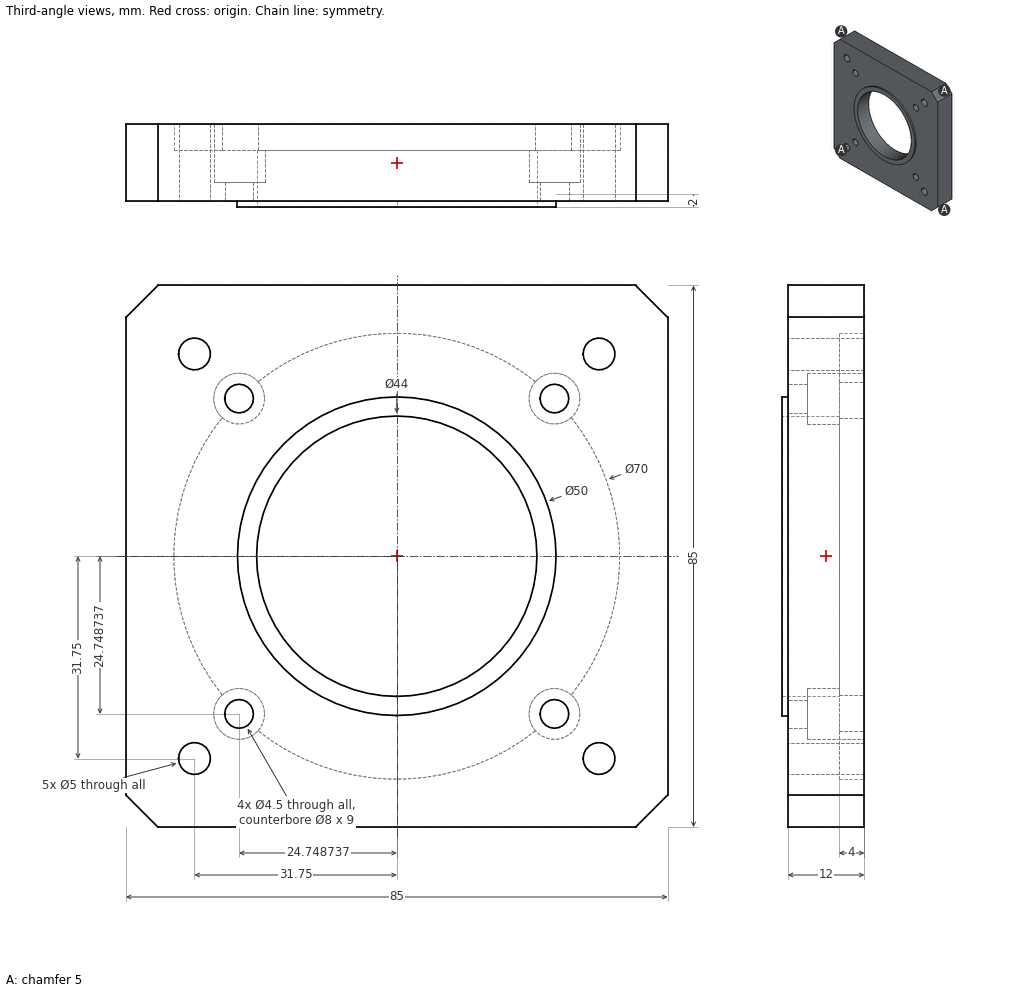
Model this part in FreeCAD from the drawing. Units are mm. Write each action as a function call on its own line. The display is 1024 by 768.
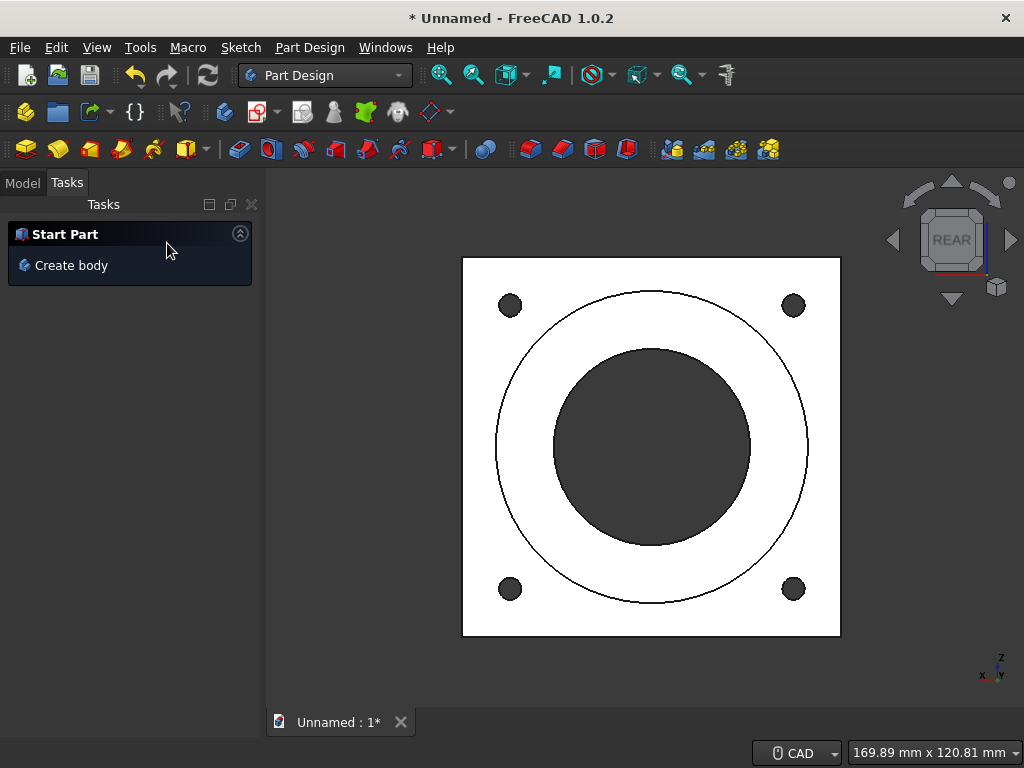
key(0)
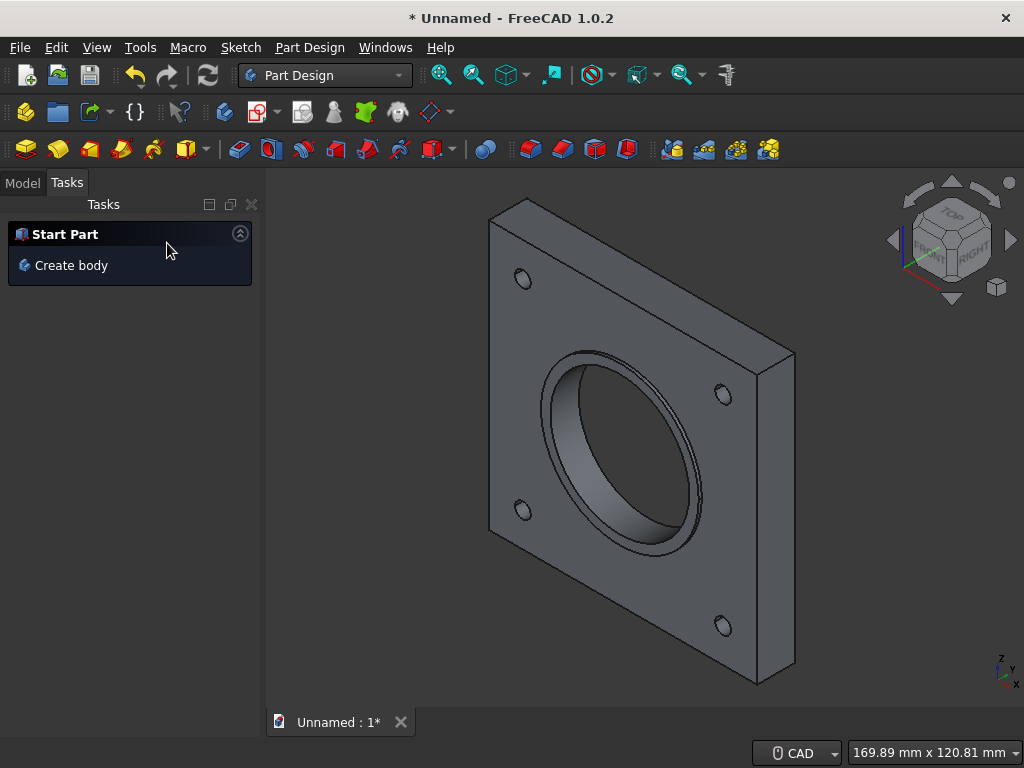
click(776, 363)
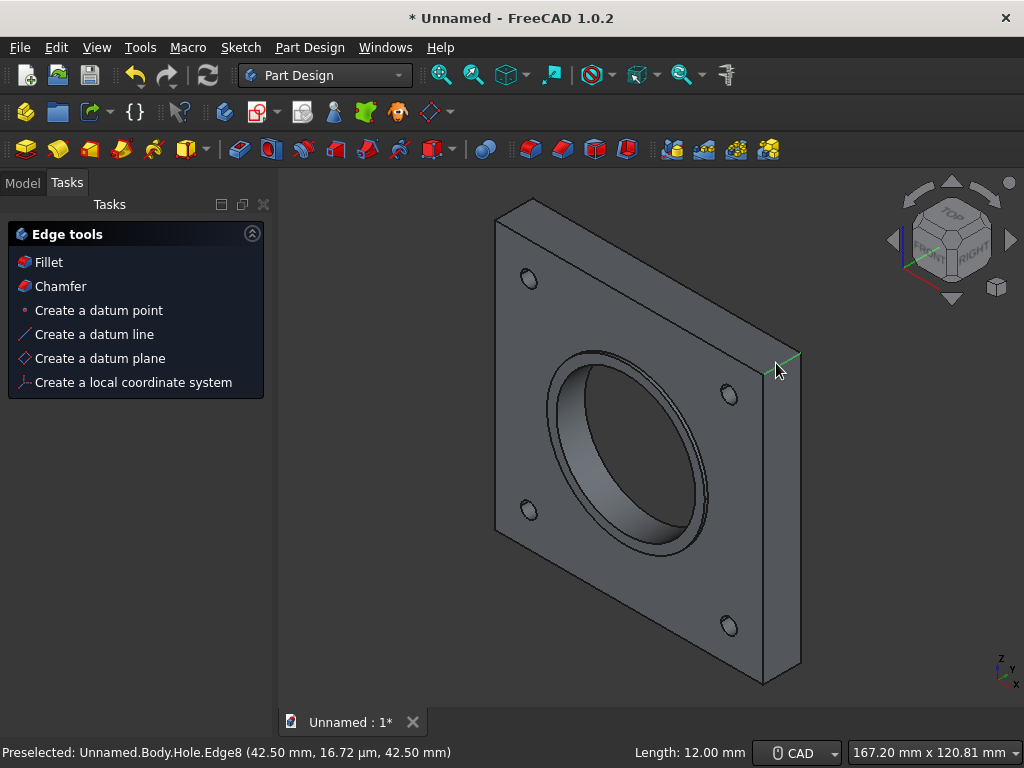
key(2)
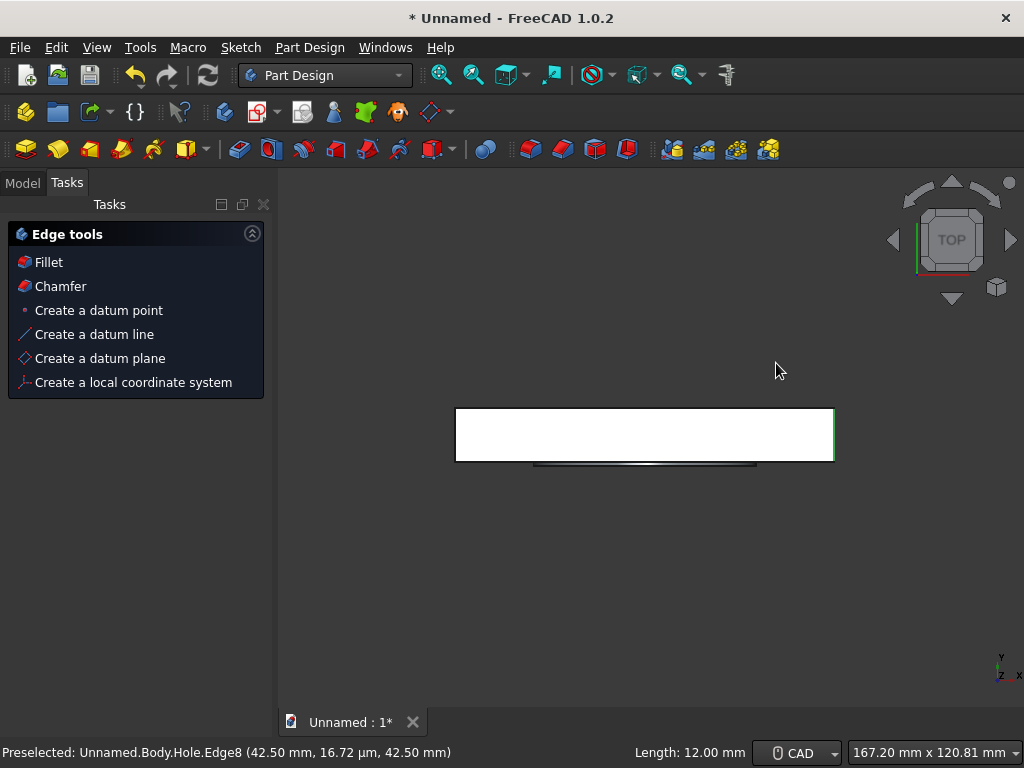
click(455, 434, ctrl)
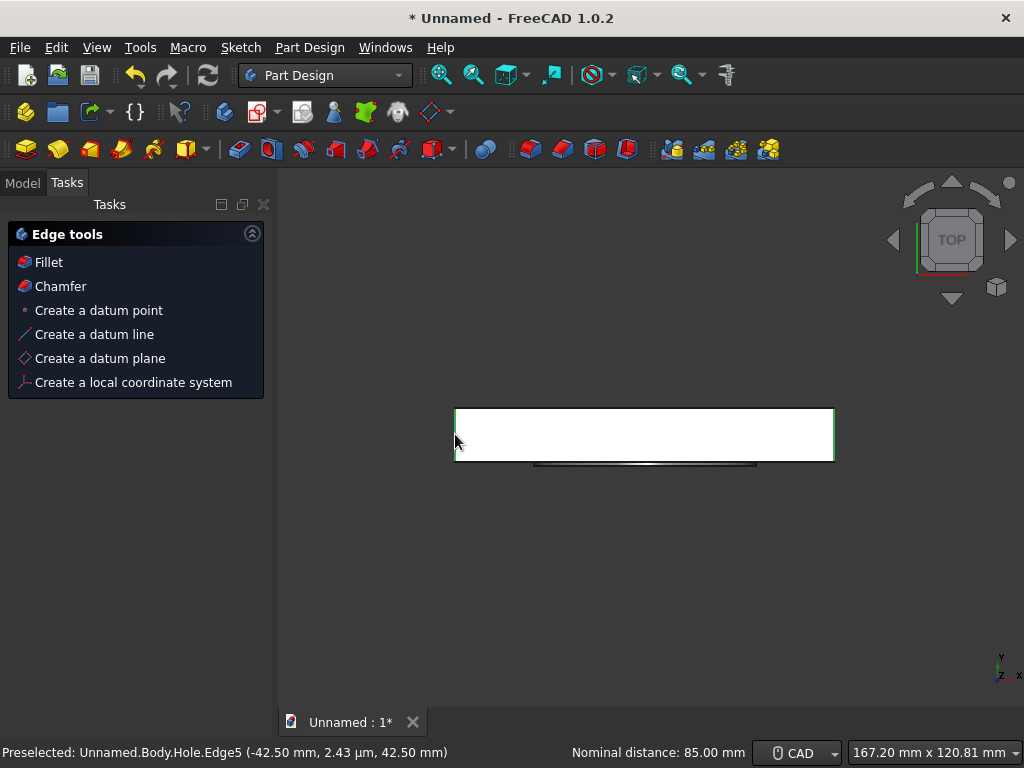
key(1)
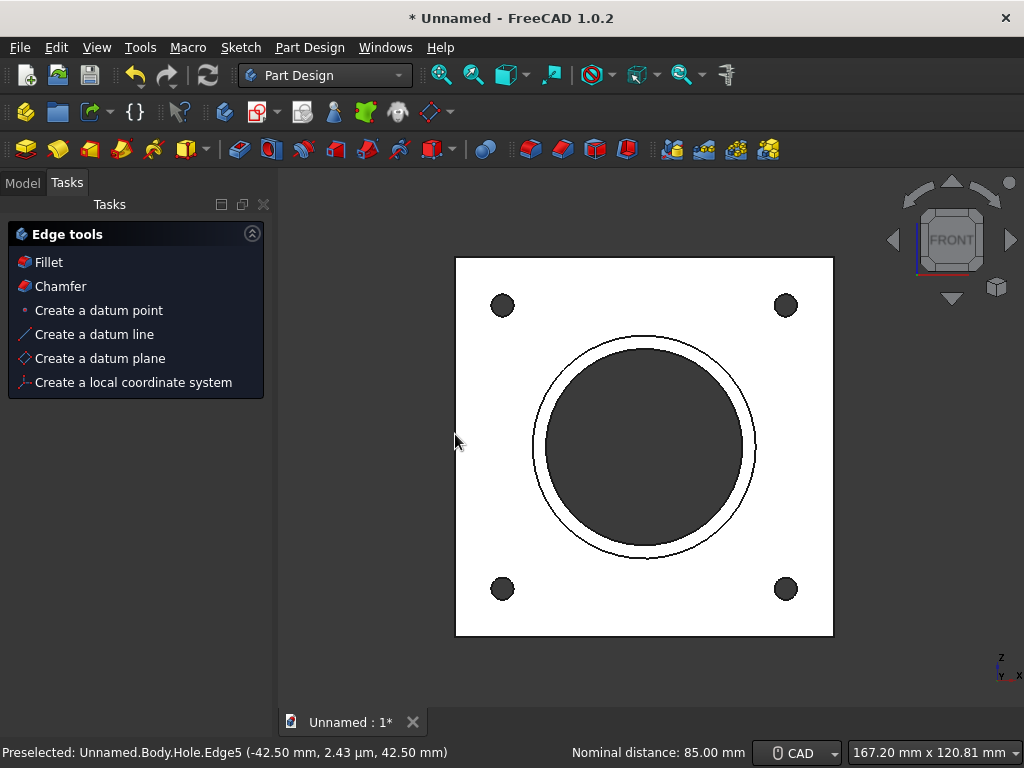
key(3)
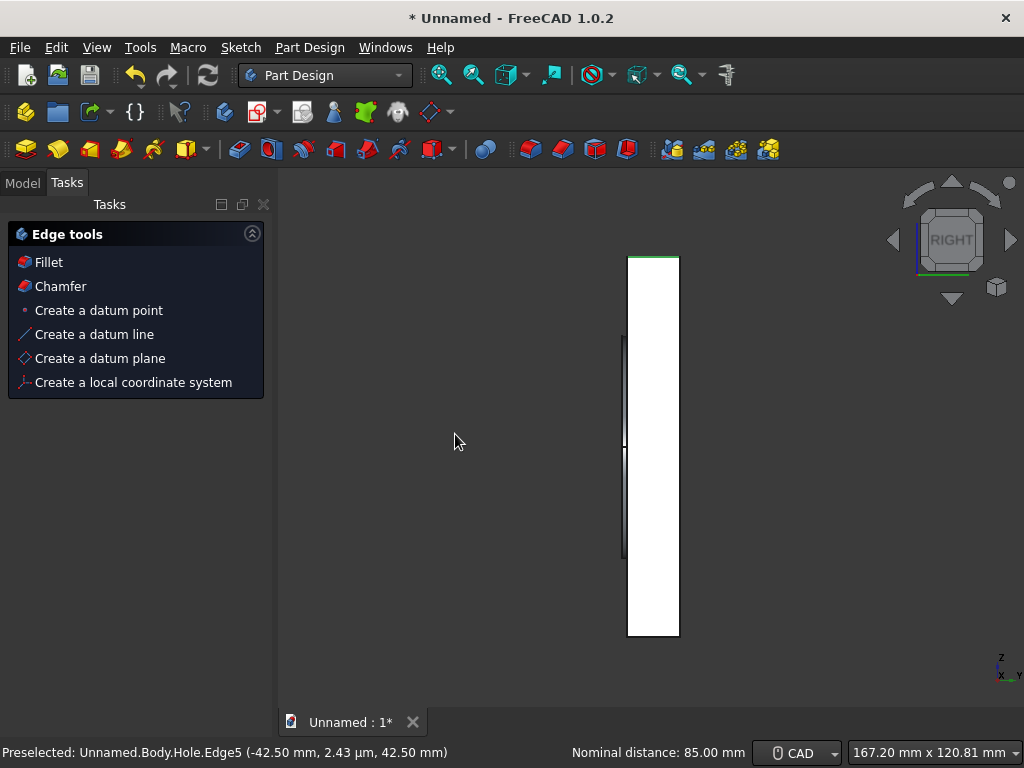
click(653, 636, ctrl)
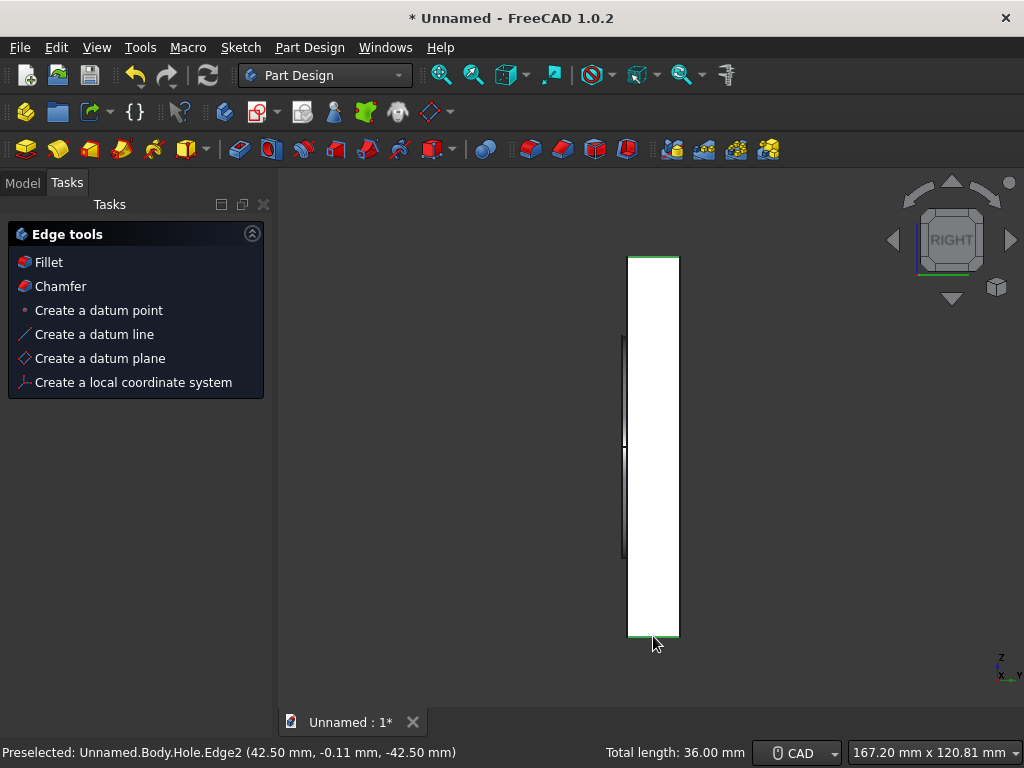
key(5)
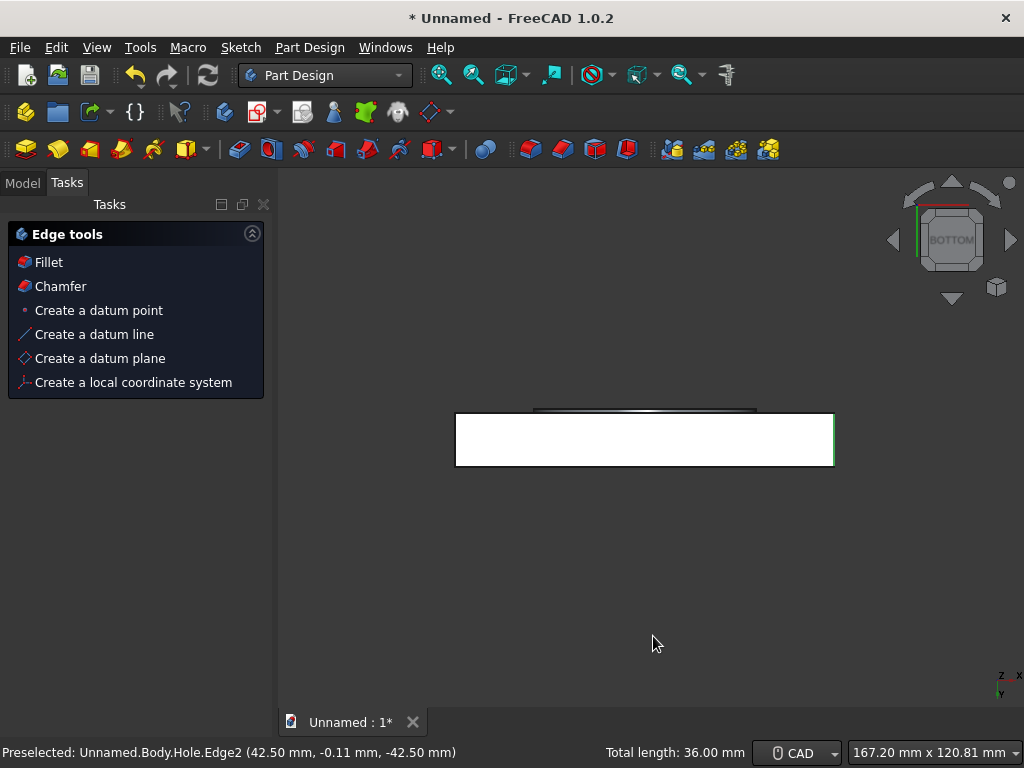
click(455, 439, ctrl)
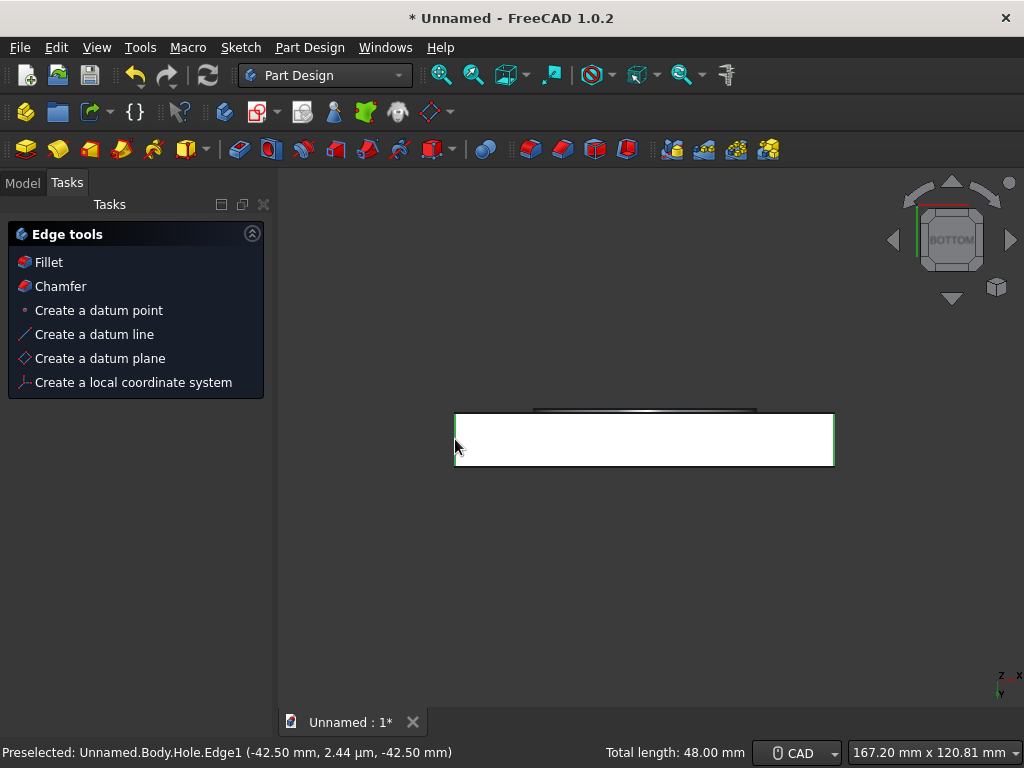
click(564, 150)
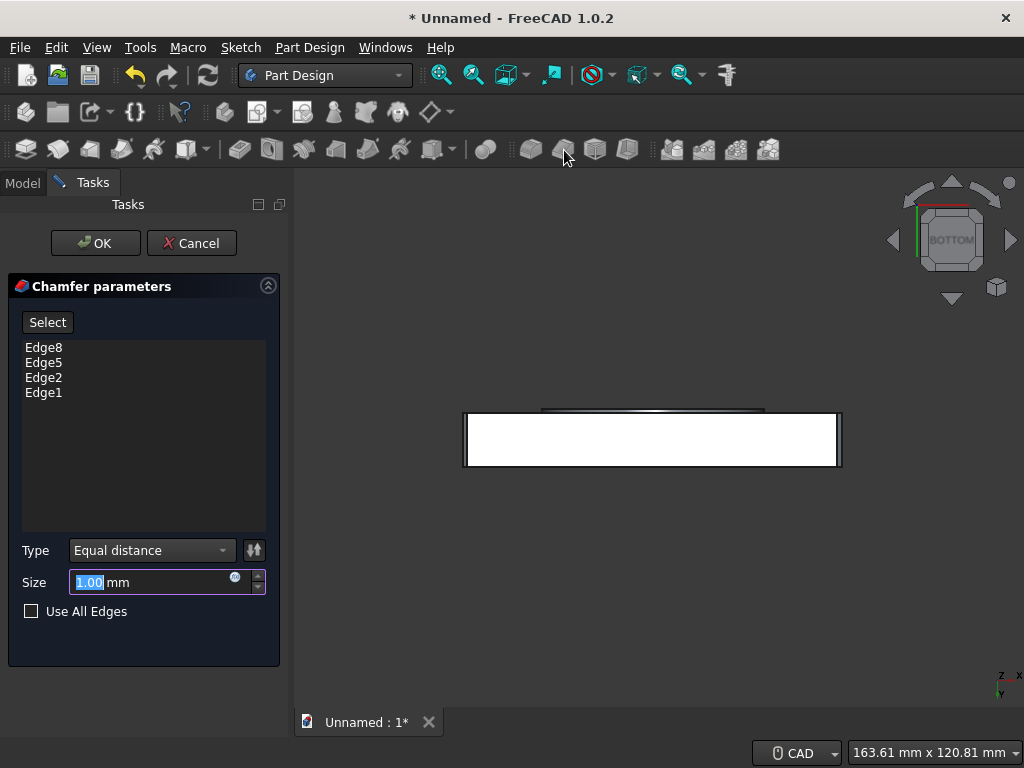
text(5)
key(Tab)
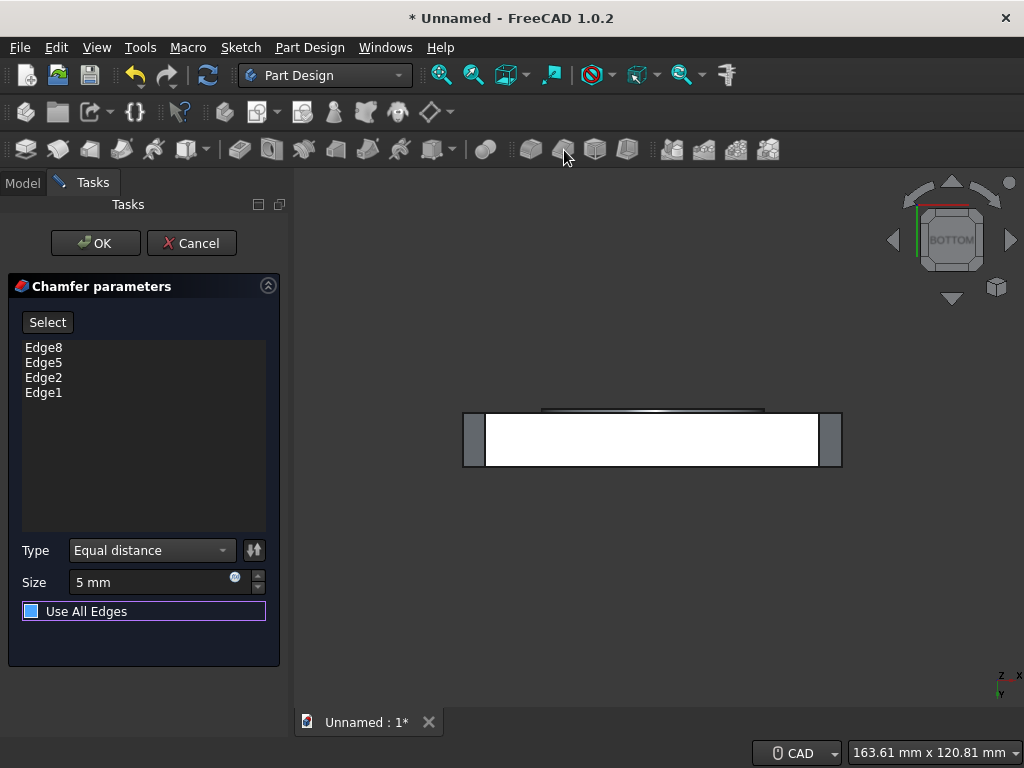
click(96, 243)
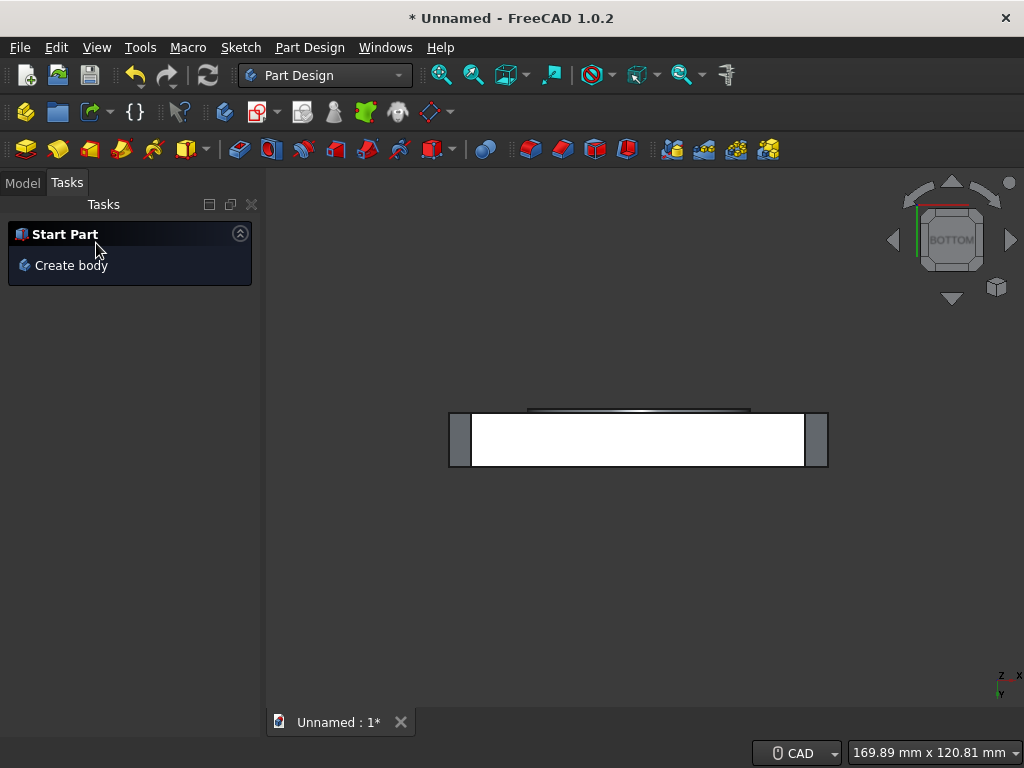
key(4)